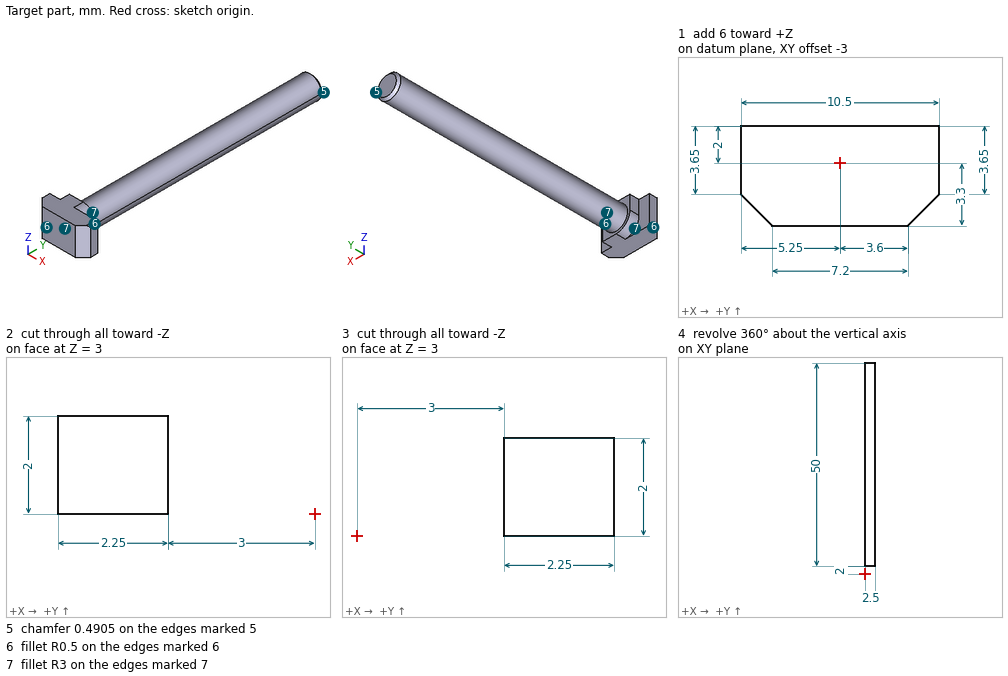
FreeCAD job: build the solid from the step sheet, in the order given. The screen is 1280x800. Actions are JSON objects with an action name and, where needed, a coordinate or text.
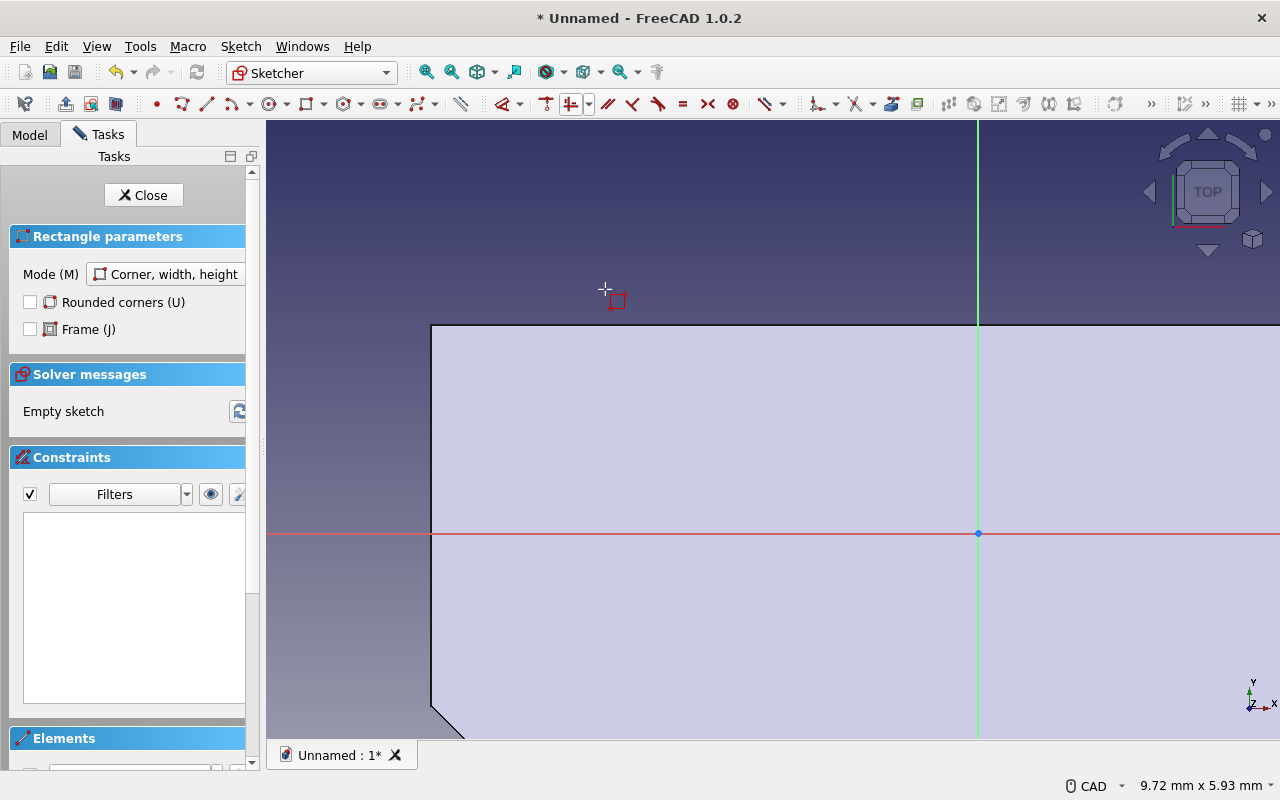
{"action": "left_click", "coordinate": [431, 325]}
{"action": "left_click", "coordinate": [665, 534]}
{"action": "key", "text": "Escape"}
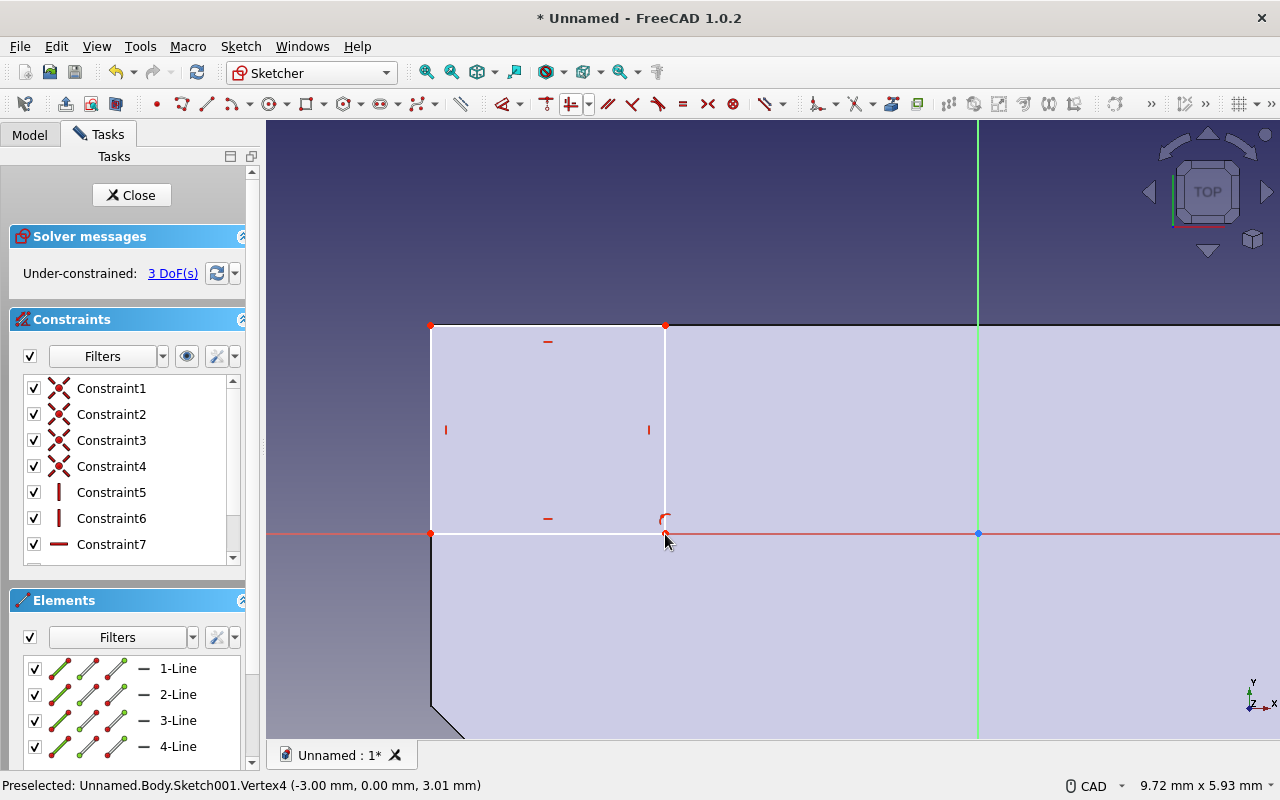
{"action": "key", "text": "d"}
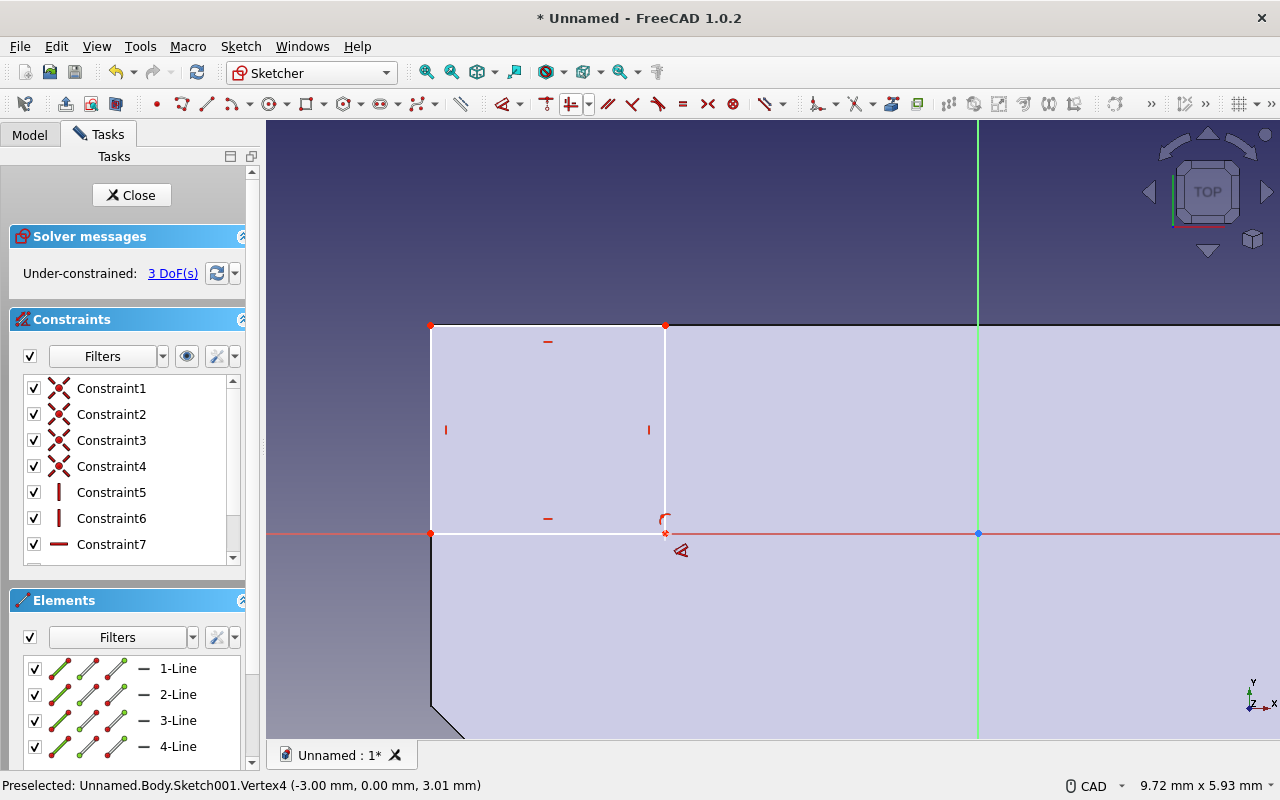
{"action": "left_click", "coordinate": [431, 388]}
{"action": "left_click", "coordinate": [397, 430]}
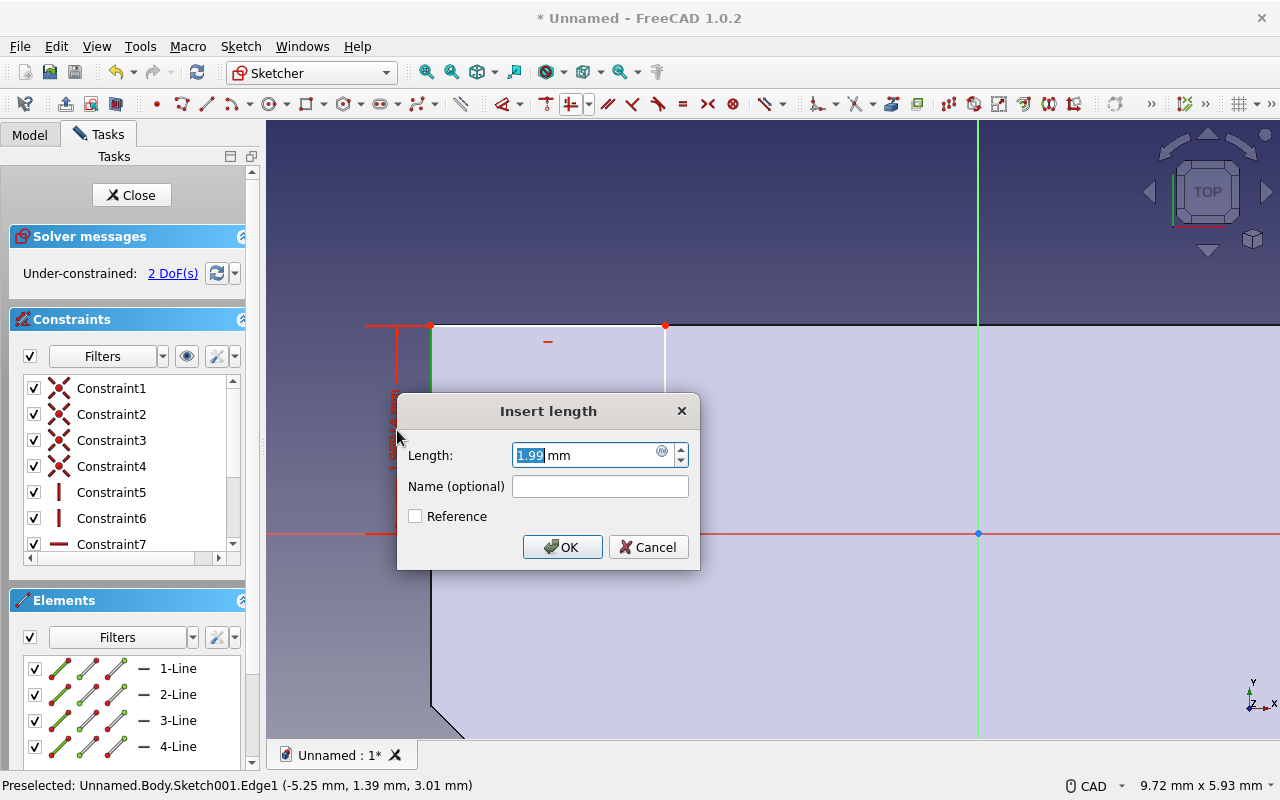
{"action": "type", "text": "2"}
{"action": "key", "text": "Return"}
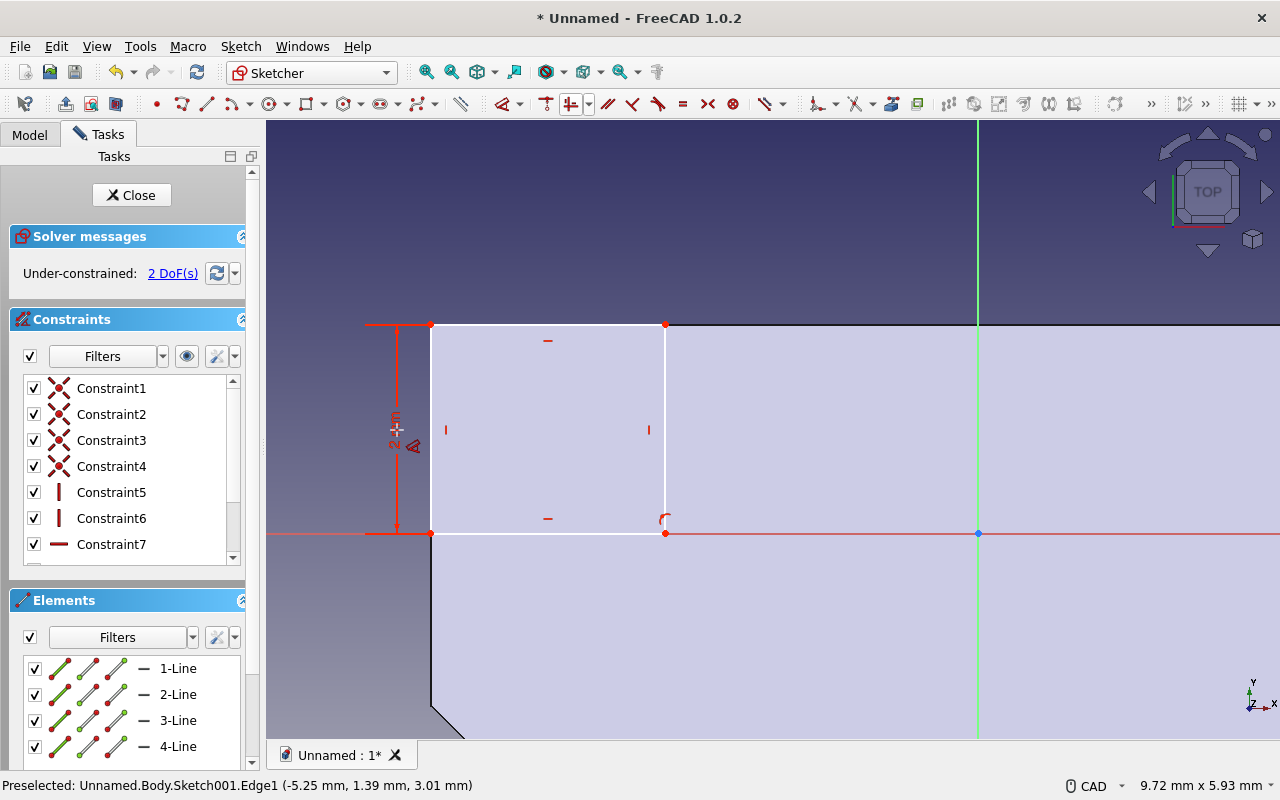
{"action": "left_click", "coordinate": [665, 534]}
{"action": "left_click", "coordinate": [822, 568]}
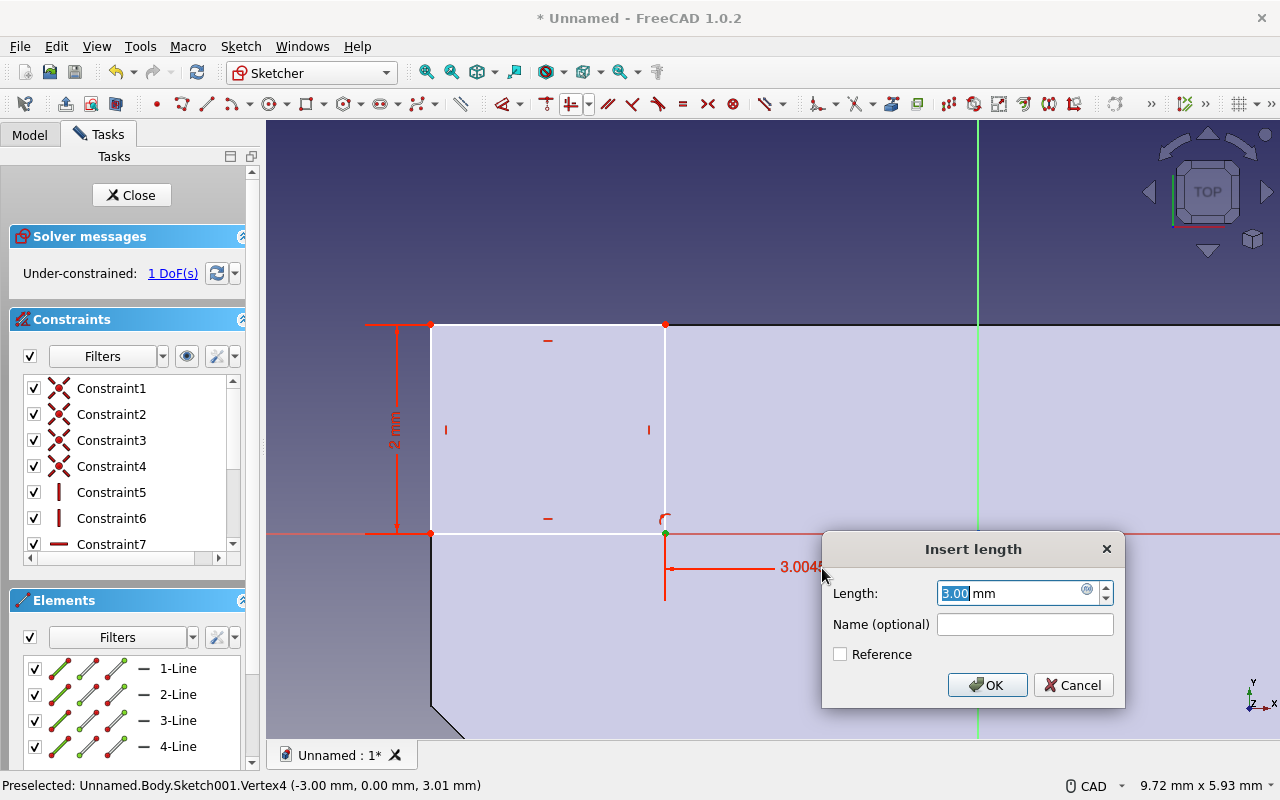
{"action": "type", "text": "3"}
{"action": "key", "text": "Return"}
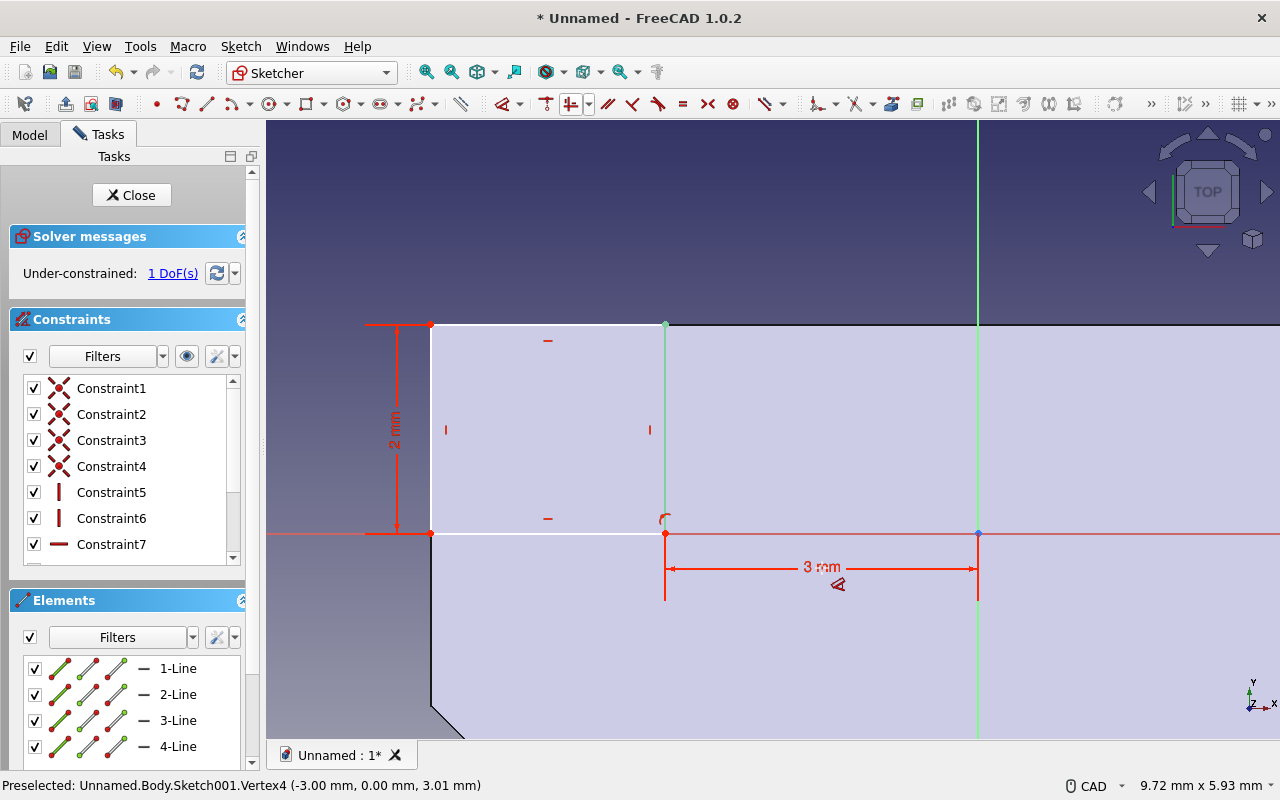
{"action": "left_click", "coordinate": [501, 534]}
{"action": "left_click", "coordinate": [548, 568]}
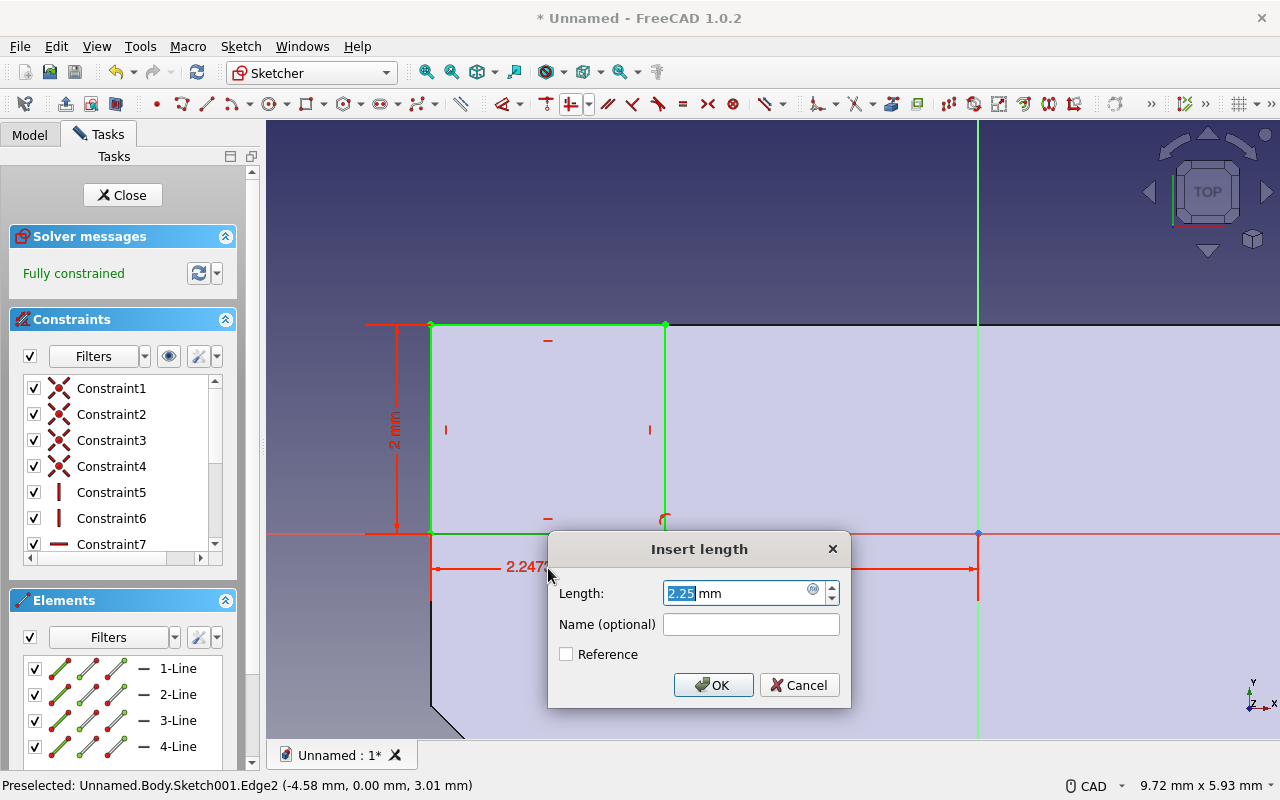
{"action": "type", "text": "2.25"}
{"action": "key", "text": "Return"}
{"action": "key", "text": "Escape"}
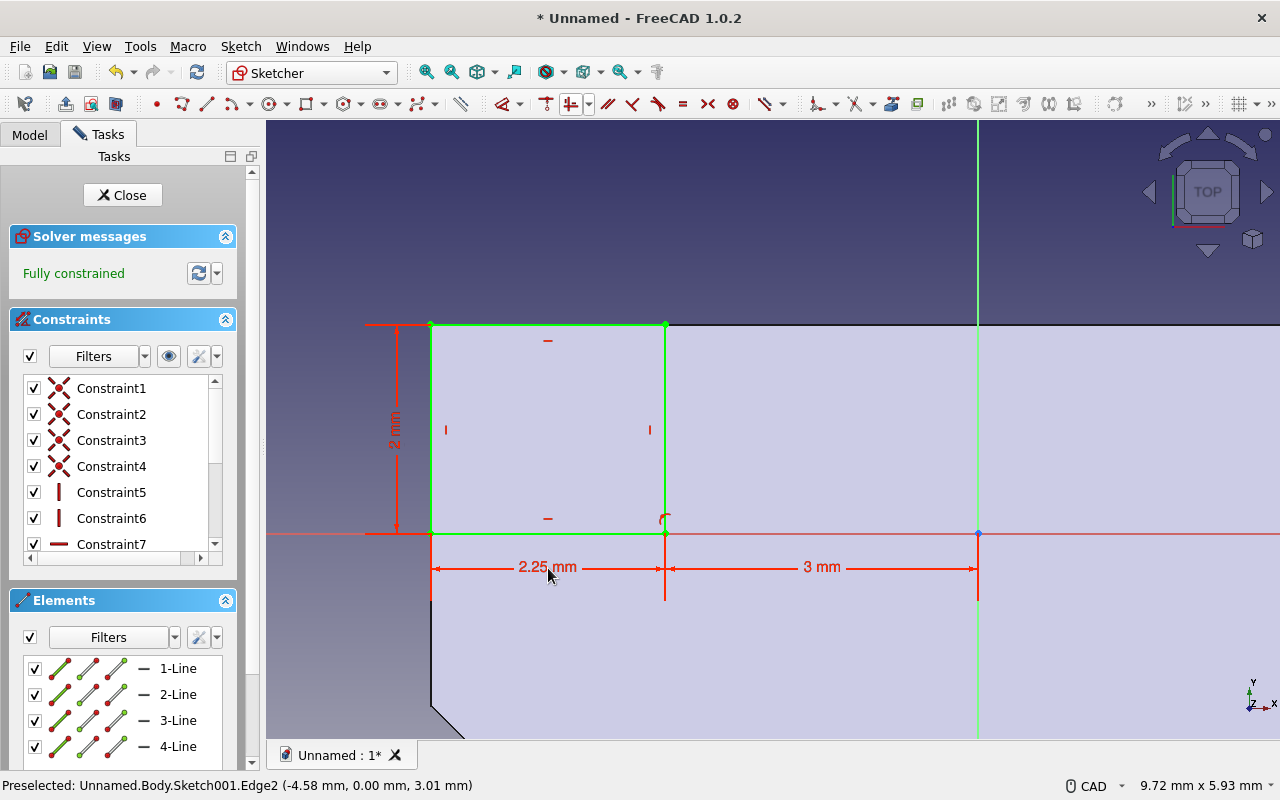
{"action": "left_click", "coordinate": [123, 195]}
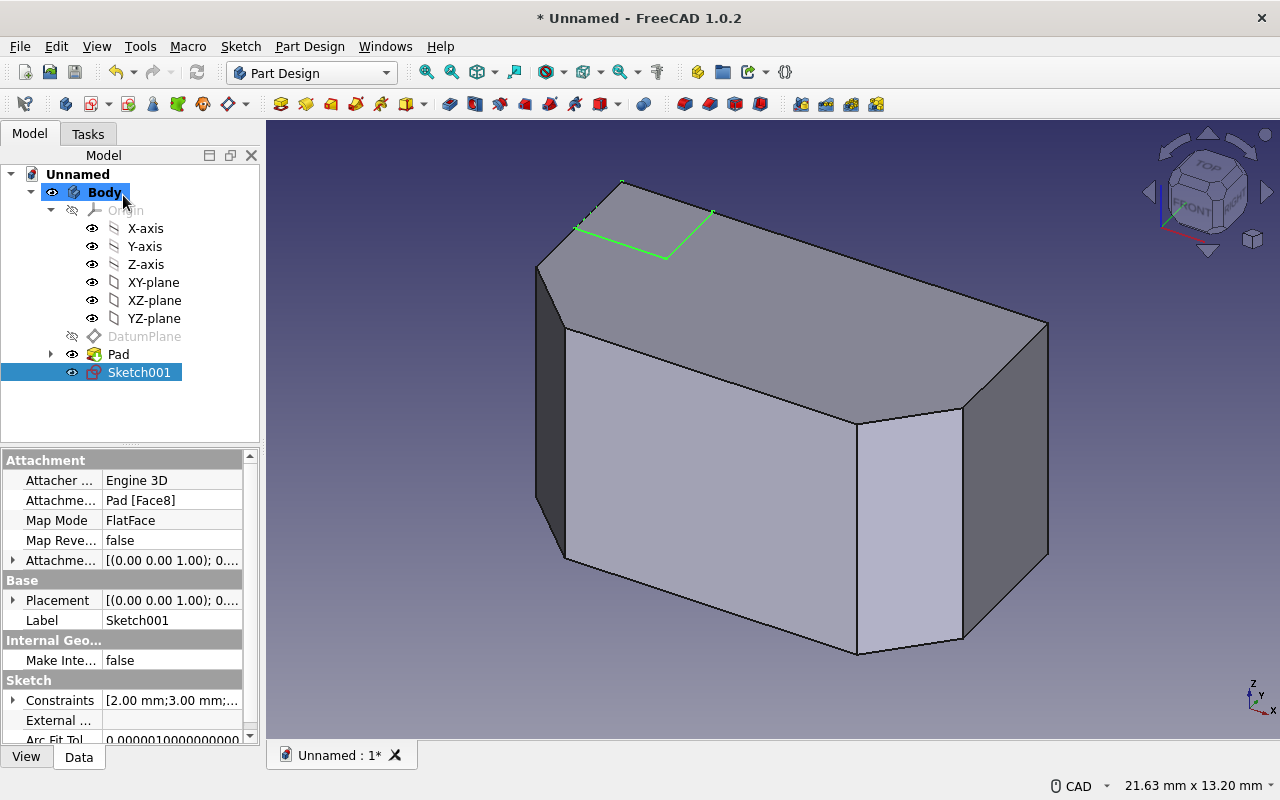
{"action": "left_click", "coordinate": [450, 104]}